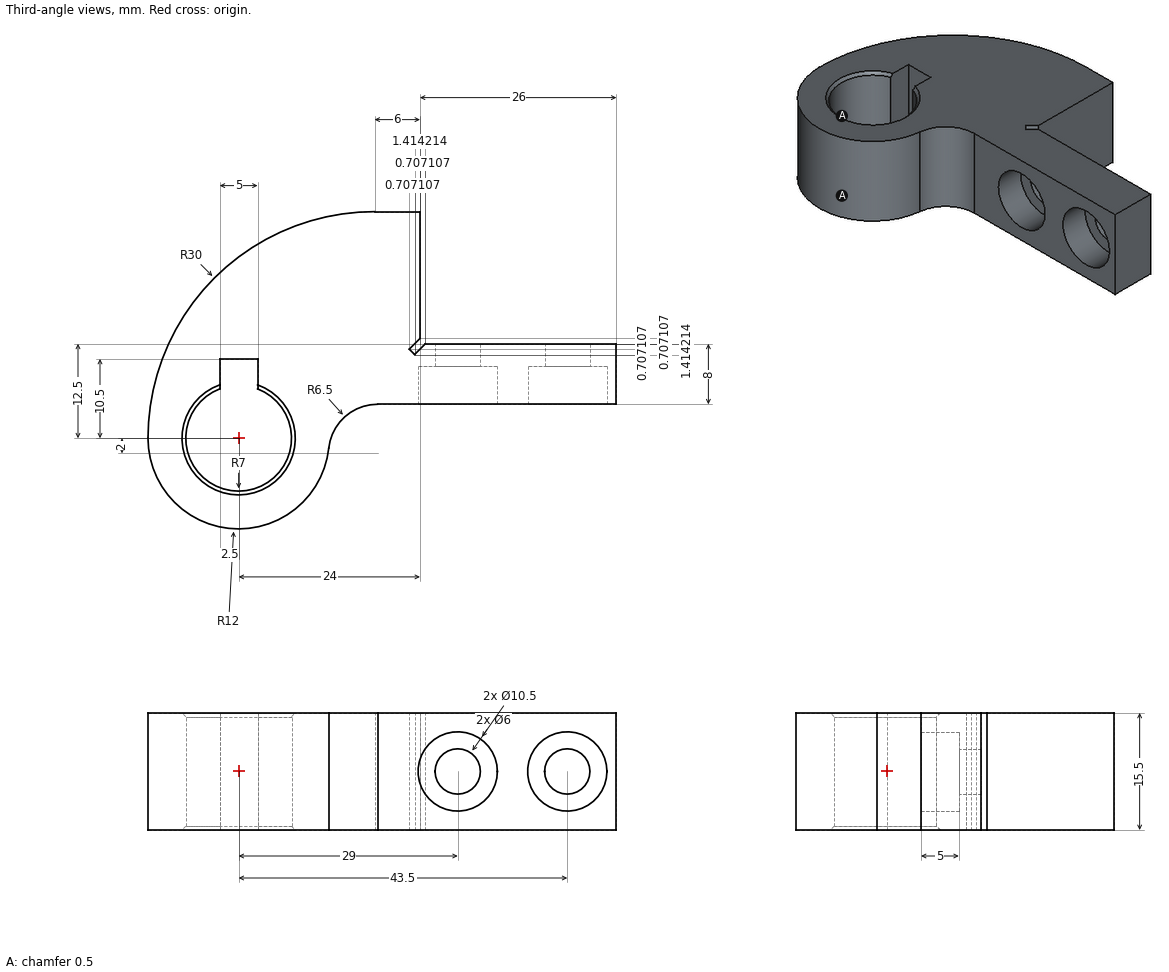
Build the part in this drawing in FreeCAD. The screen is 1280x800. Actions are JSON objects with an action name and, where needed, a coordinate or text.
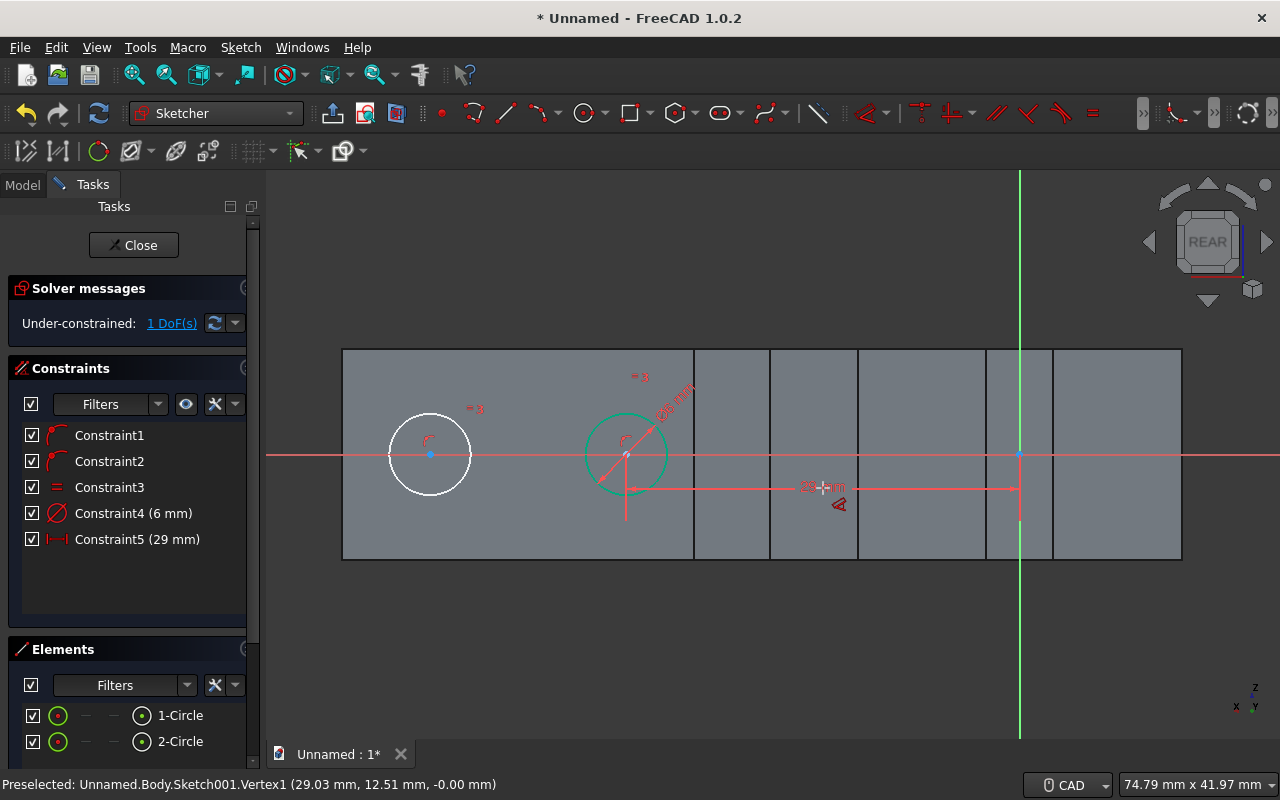
{"action": "left_click", "coordinate": [430, 454]}
{"action": "left_click", "coordinate": [725, 488]}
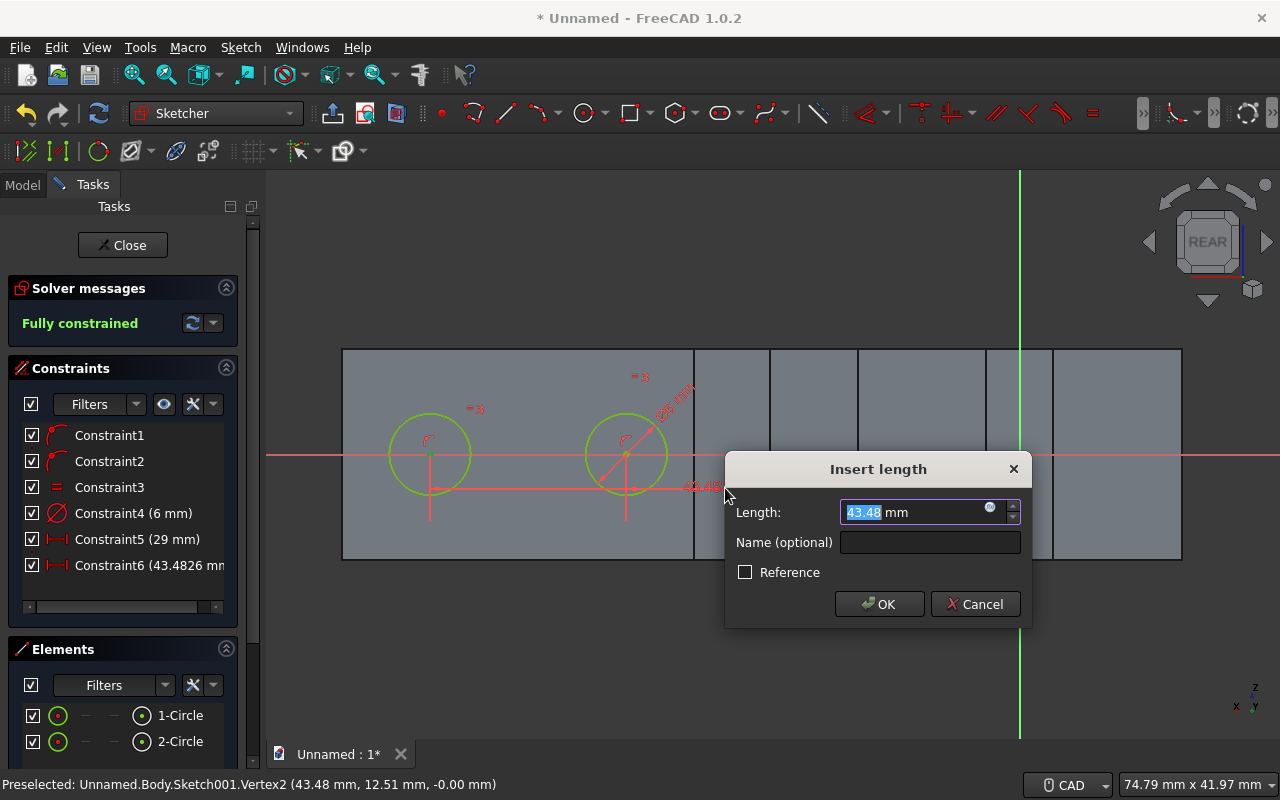
{"action": "type", "text": "43.5"}
{"action": "key", "text": "Return"}
{"action": "key", "text": "Escape"}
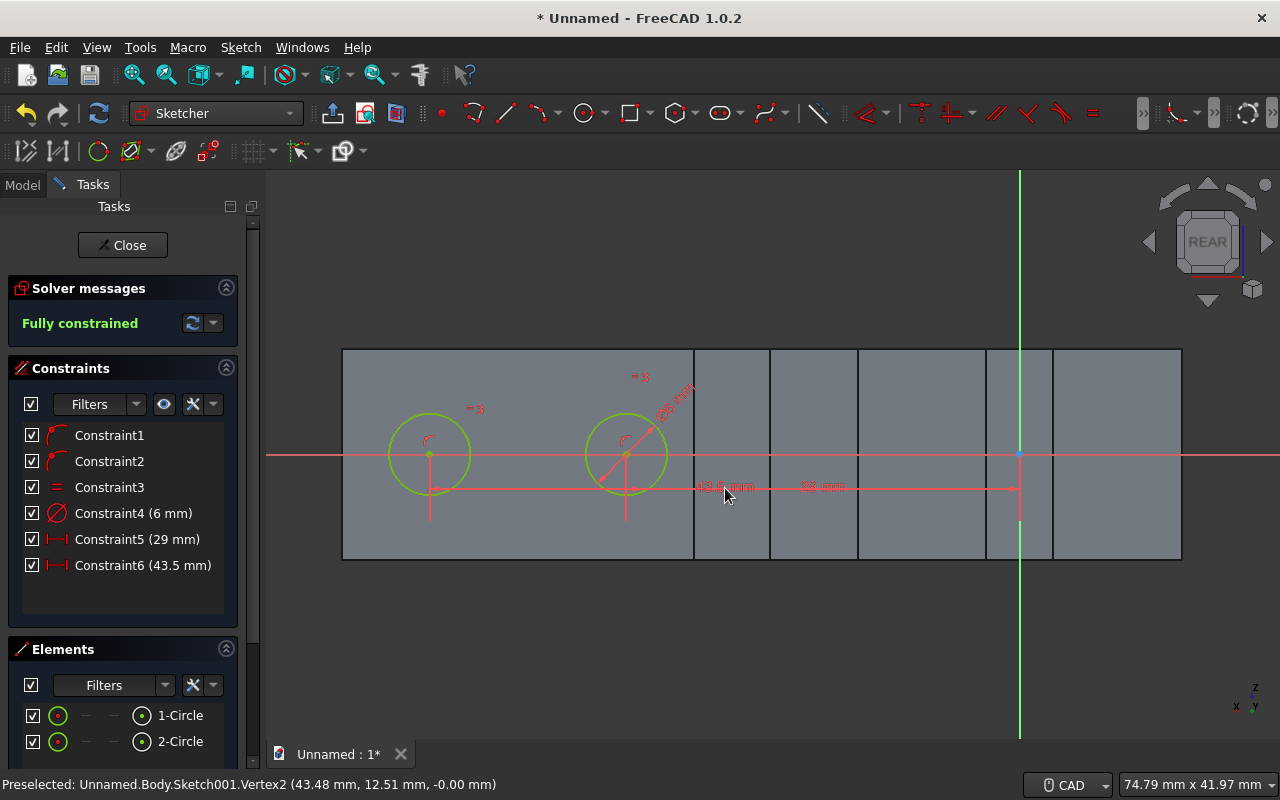
{"action": "left_click", "coordinate": [123, 245]}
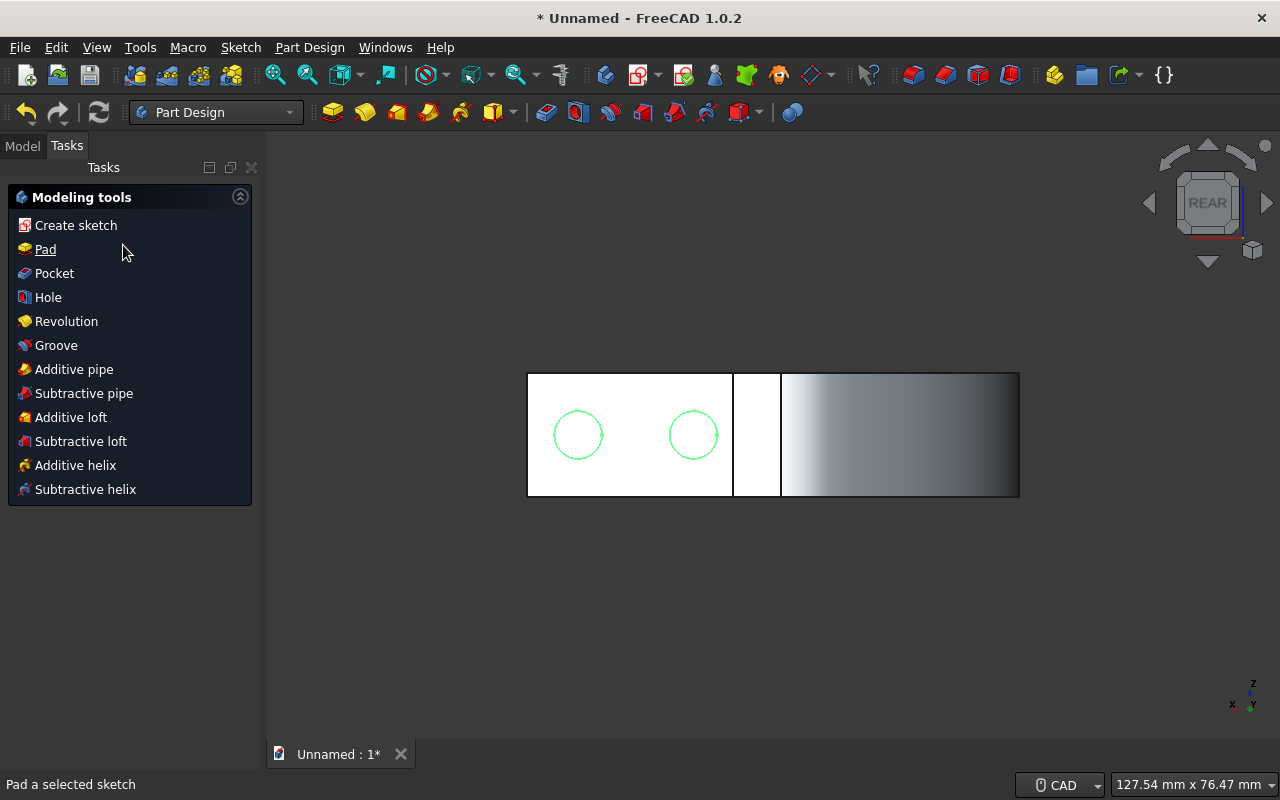
{"action": "left_click", "coordinate": [548, 112]}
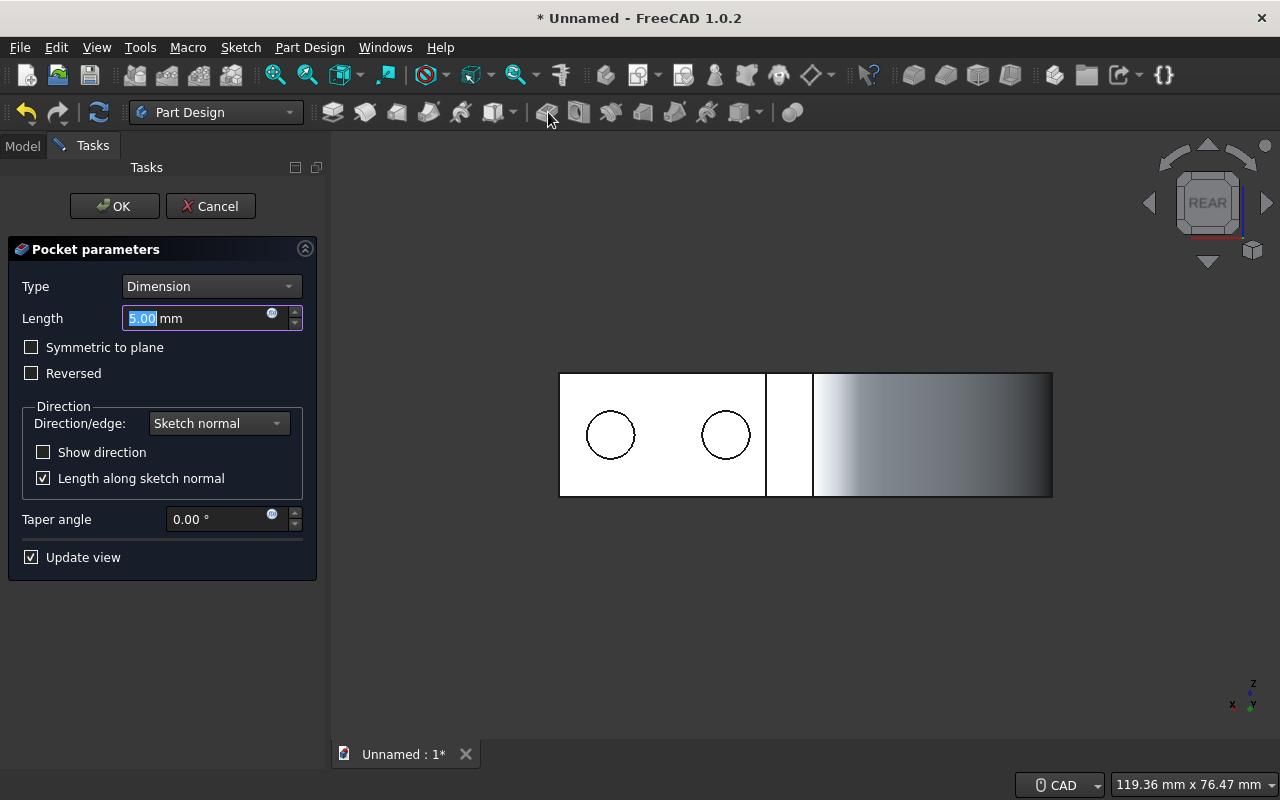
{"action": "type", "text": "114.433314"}
{"action": "key", "text": "Tab"}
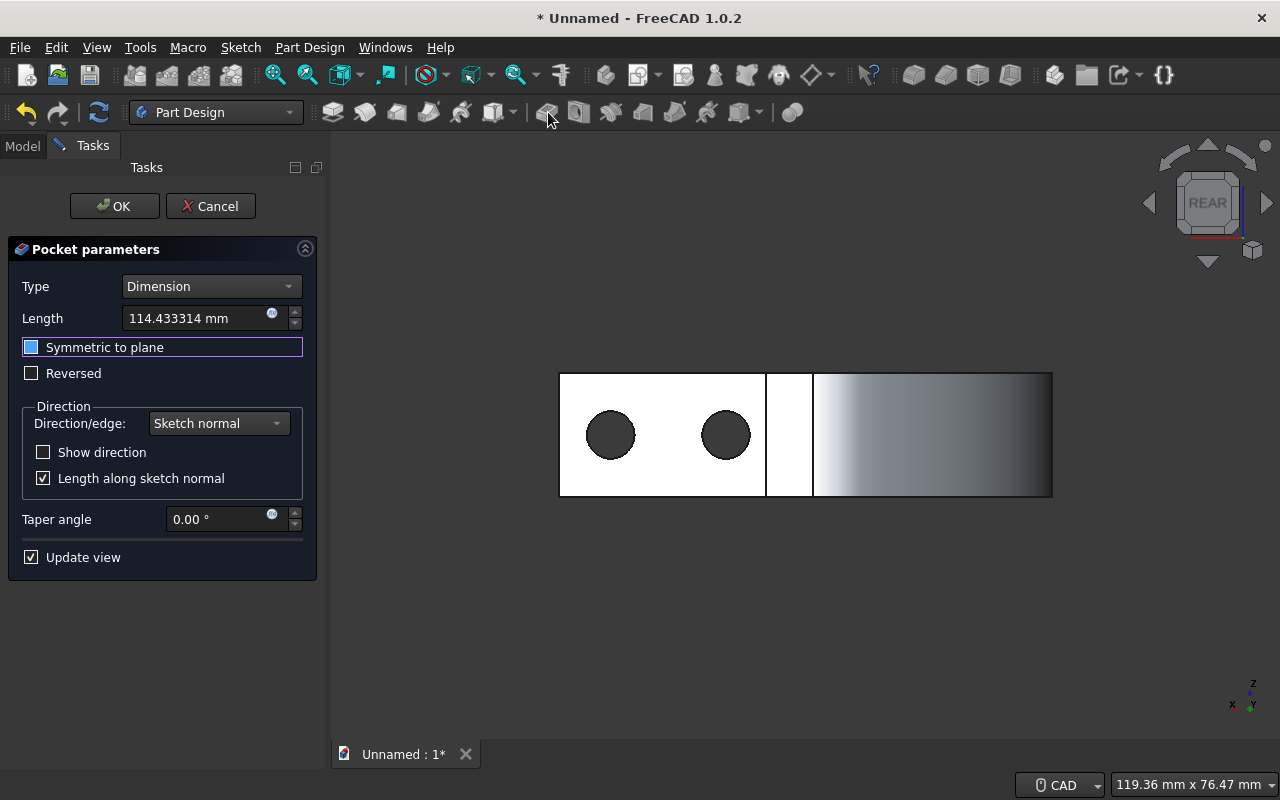
{"action": "left_click", "coordinate": [30, 347]}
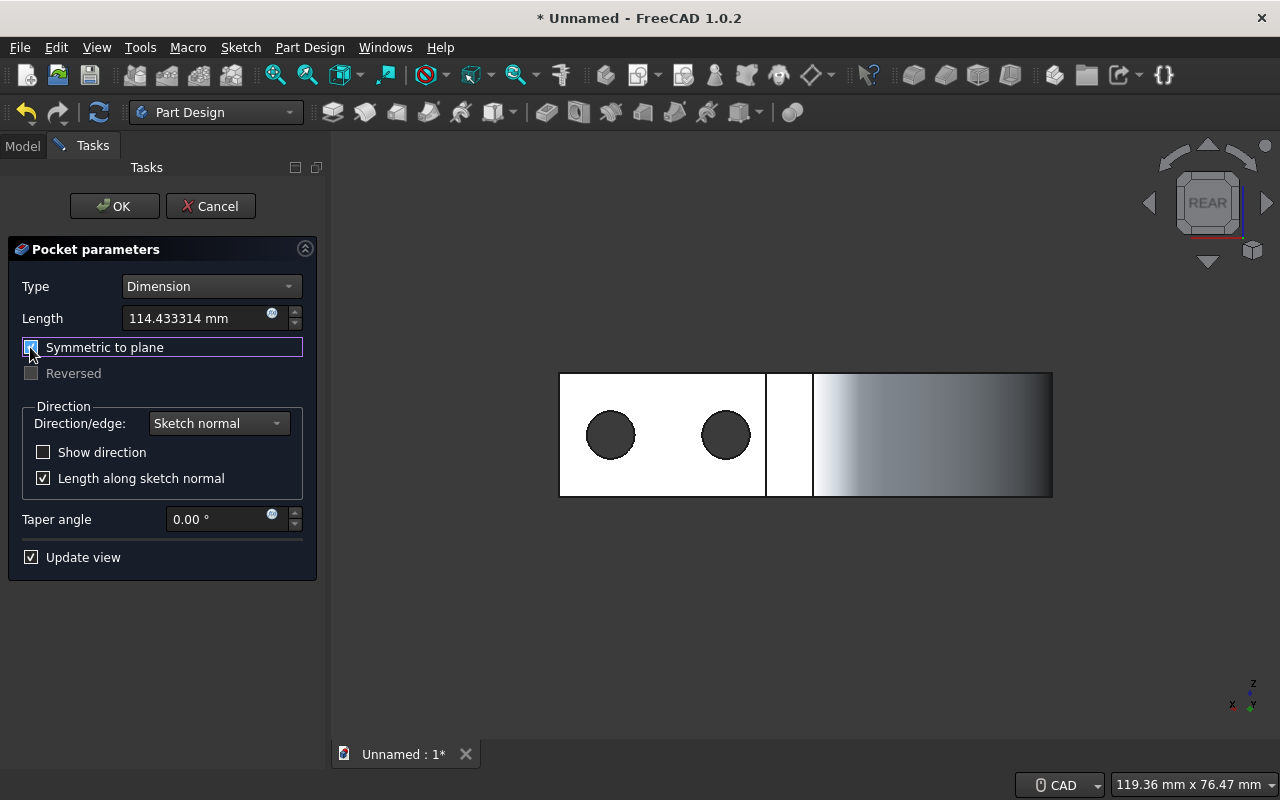
{"action": "left_click", "coordinate": [115, 206]}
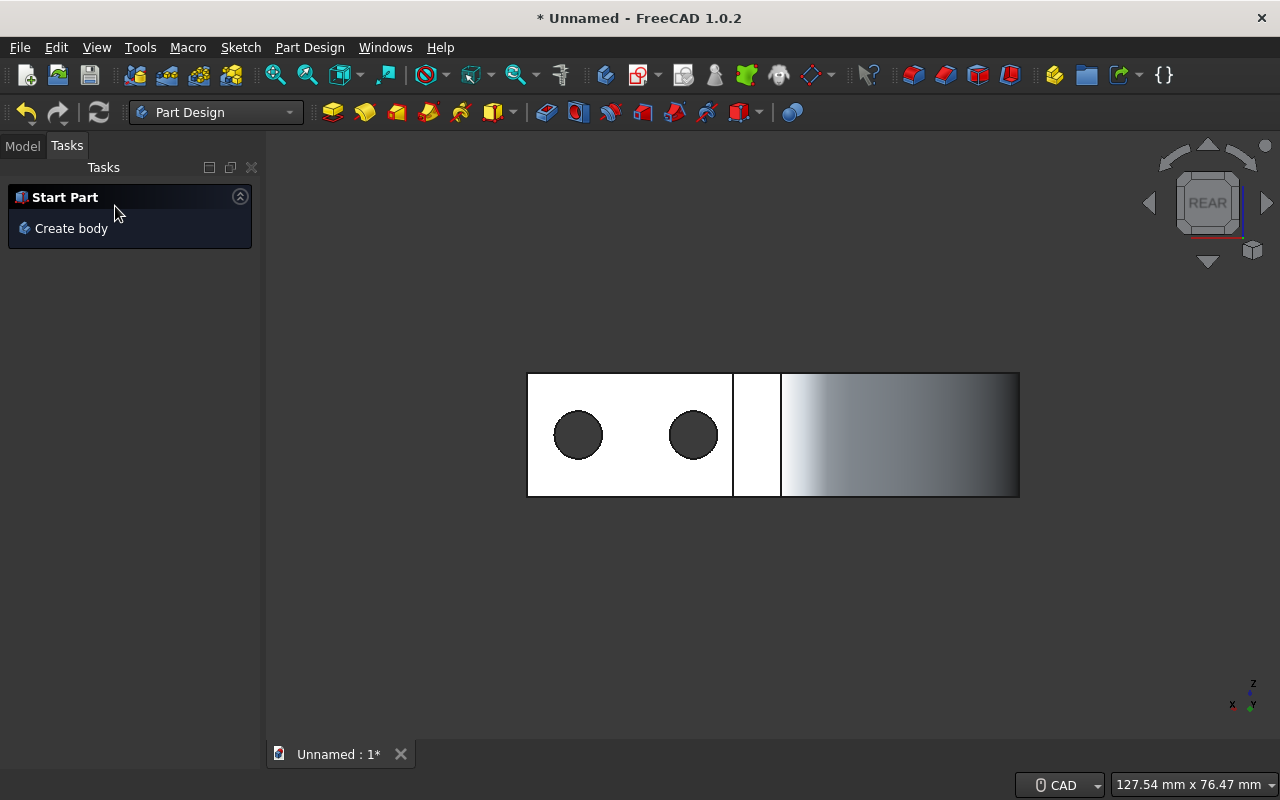
{"action": "key", "text": "0"}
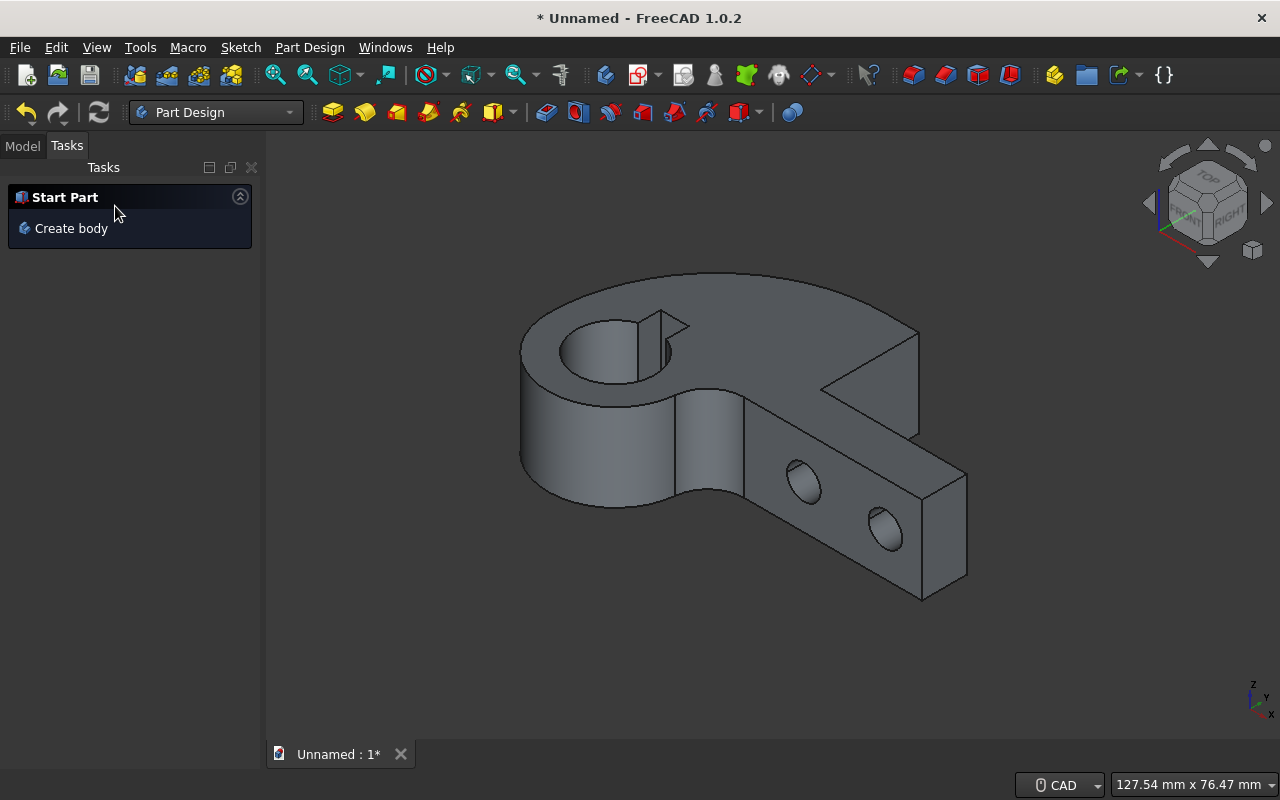
{"action": "left_click", "coordinate": [859, 484]}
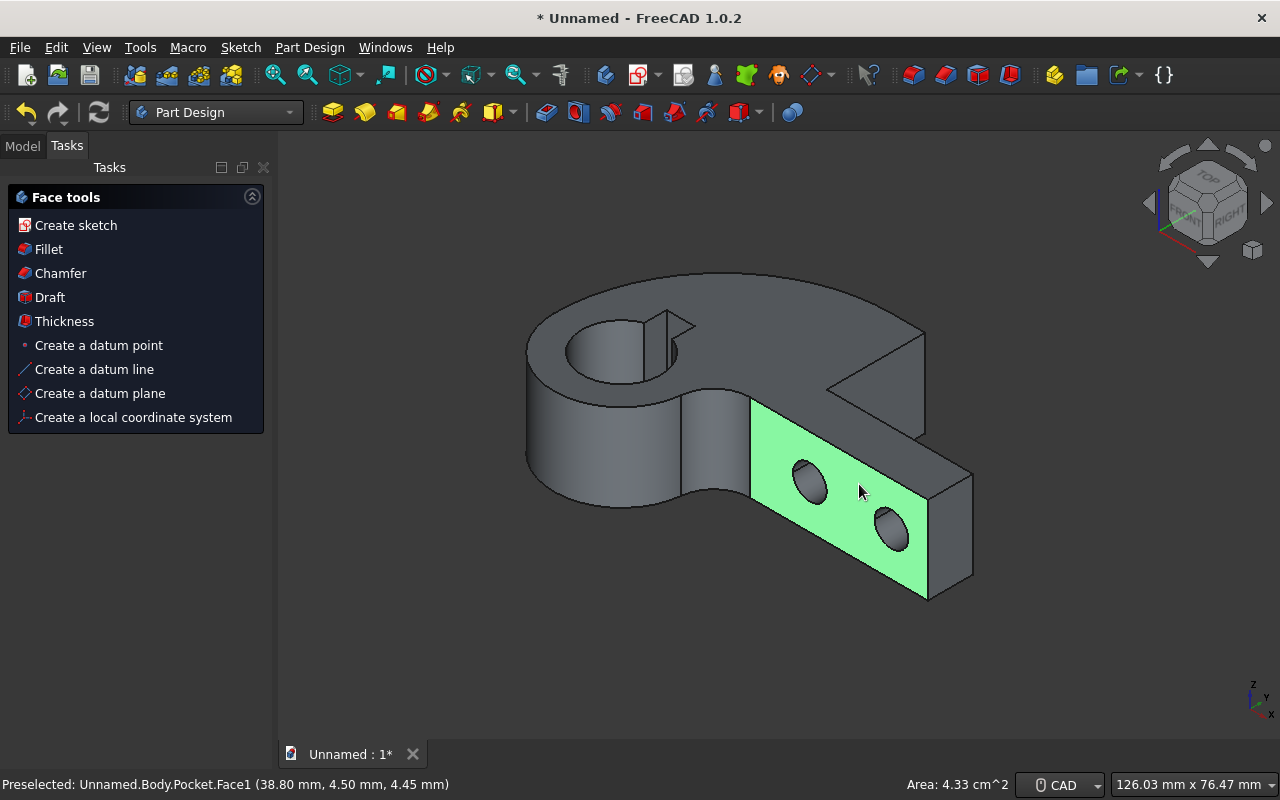
{"action": "left_click", "coordinate": [638, 76]}